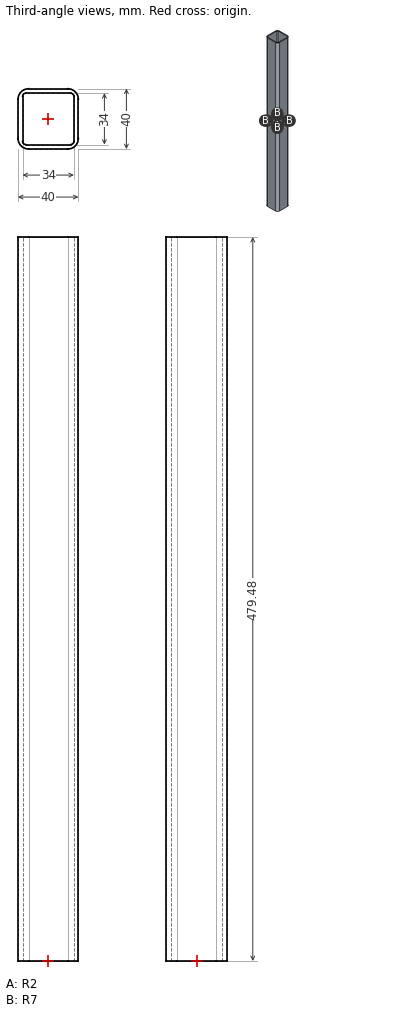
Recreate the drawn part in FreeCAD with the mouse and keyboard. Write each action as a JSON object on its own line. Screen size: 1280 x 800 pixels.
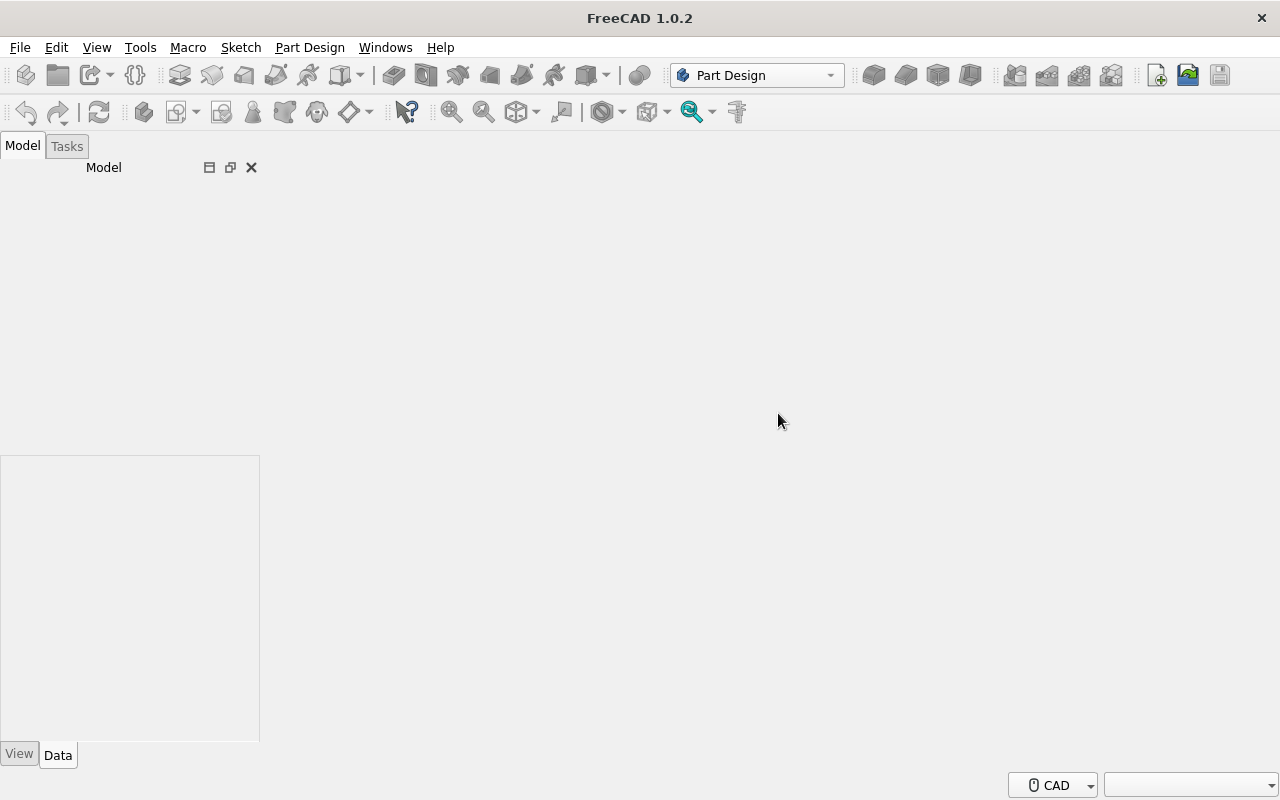
{"action": "key", "text": "ctrl+n"}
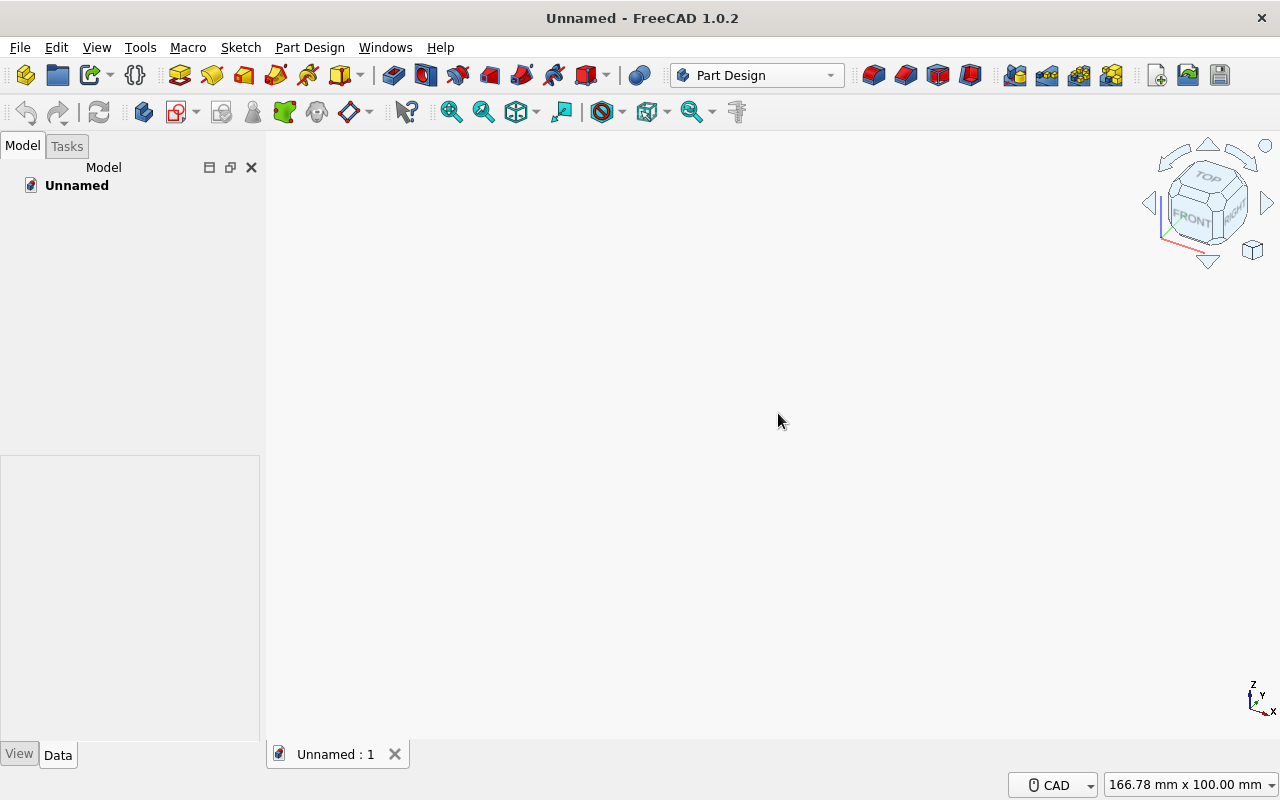
{"action": "left_click", "coordinate": [176, 112]}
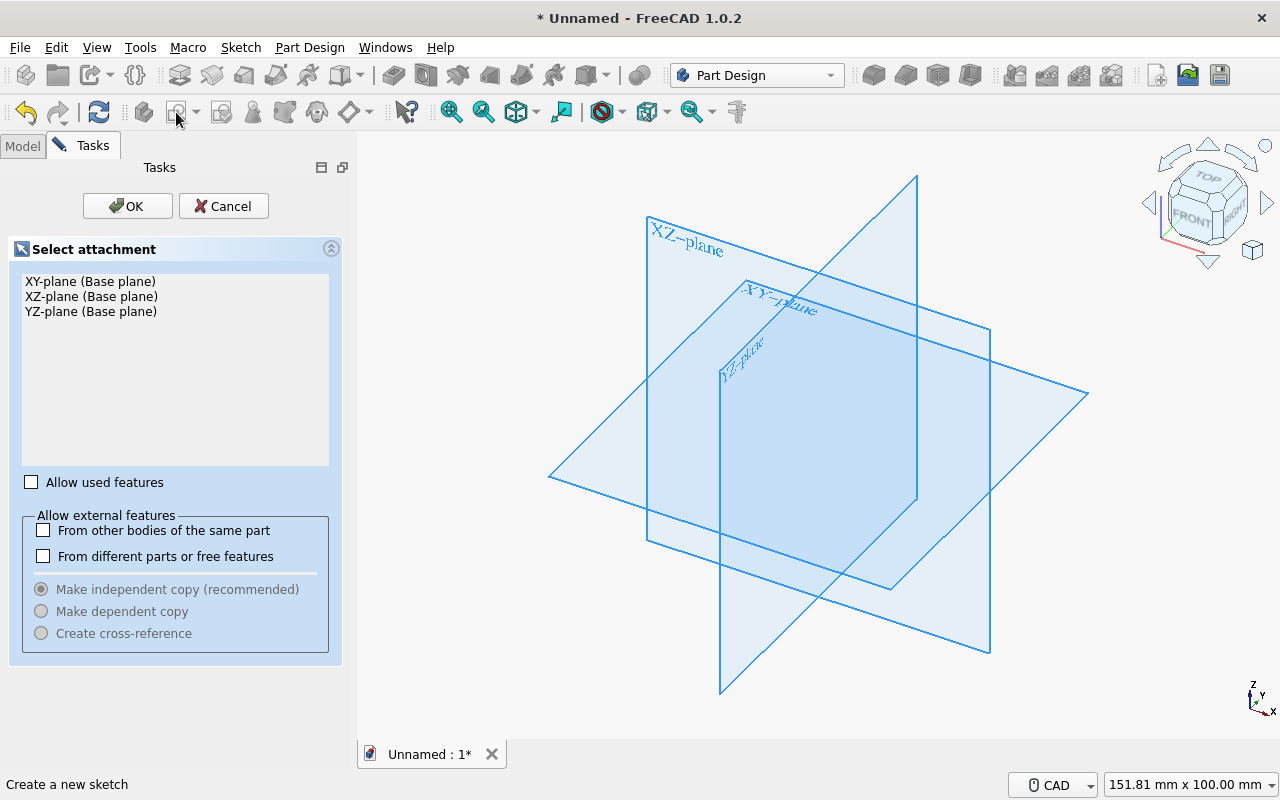
{"action": "left_click", "coordinate": [82, 282]}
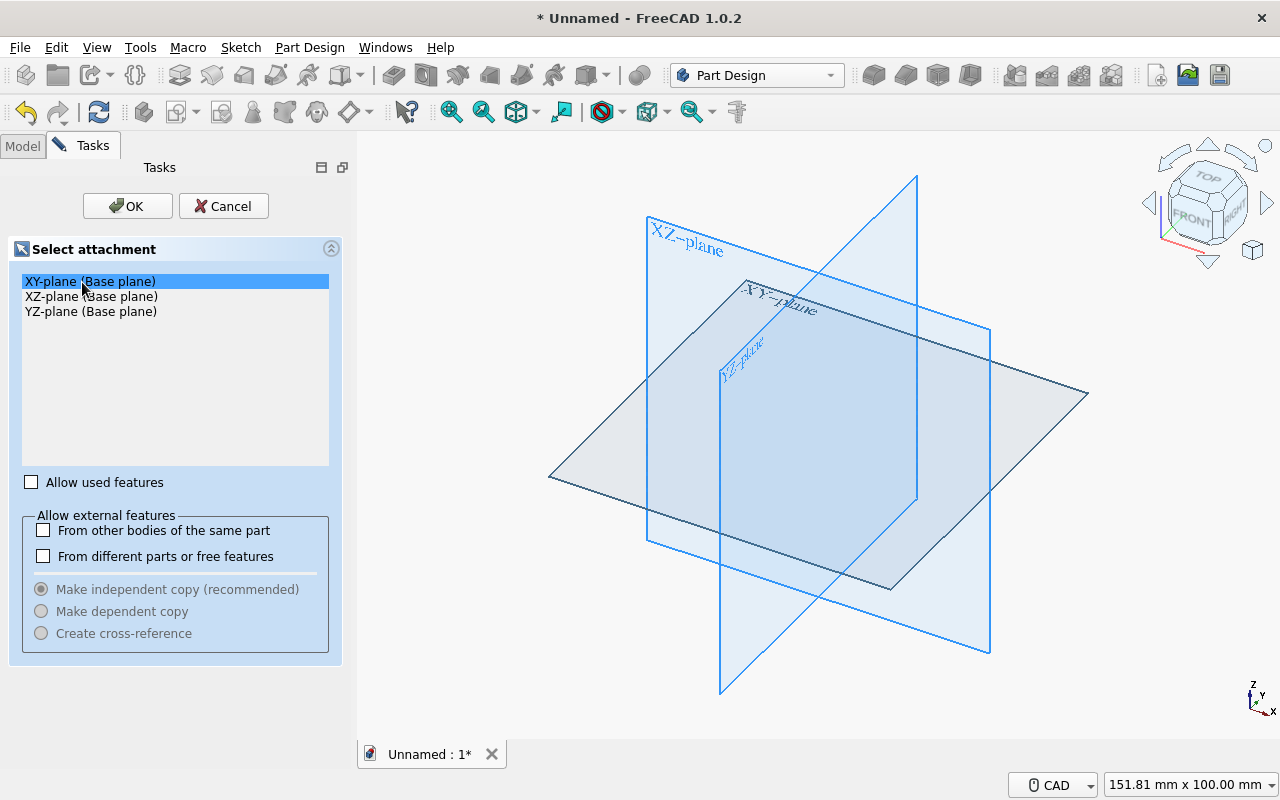
{"action": "left_click", "coordinate": [128, 206]}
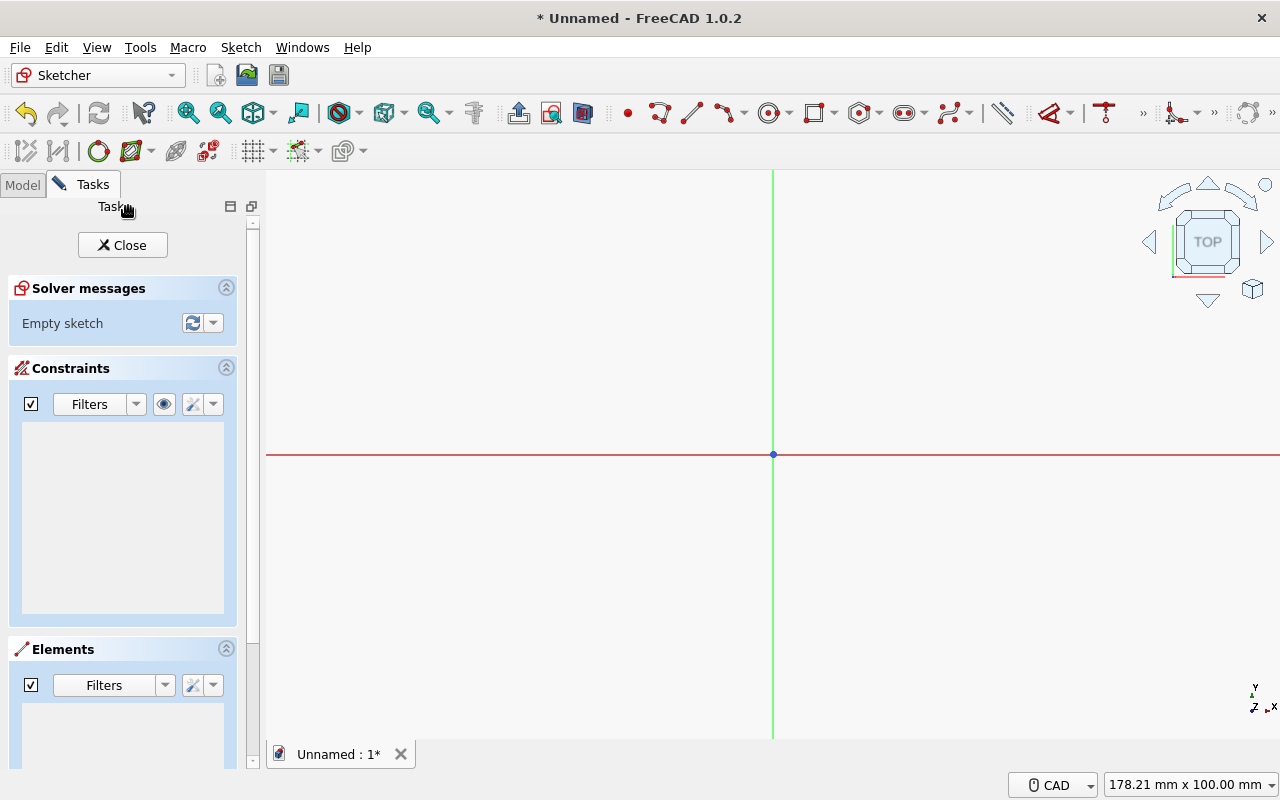
{"action": "scroll", "coordinate": [912, 455], "scroll_direction": "up", "scroll_amount": 2}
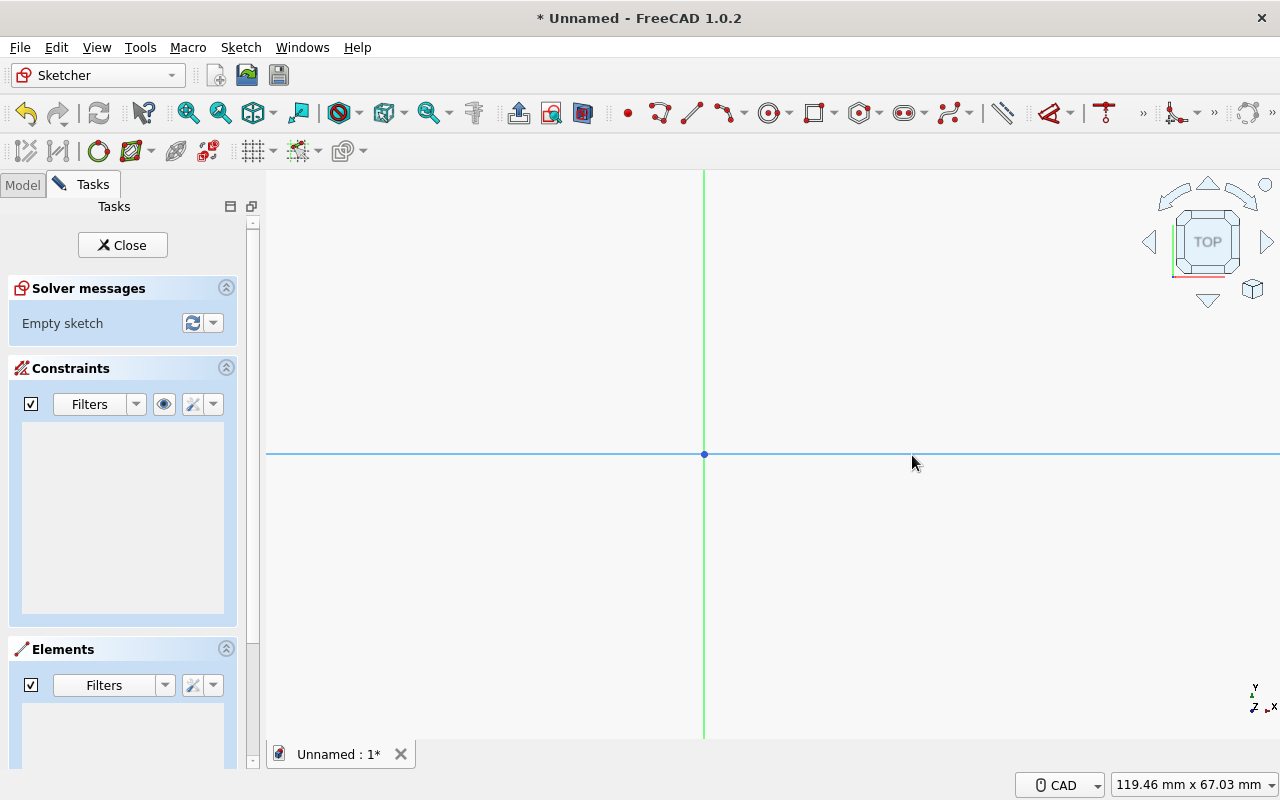
{"action": "left_click", "coordinate": [836, 114]}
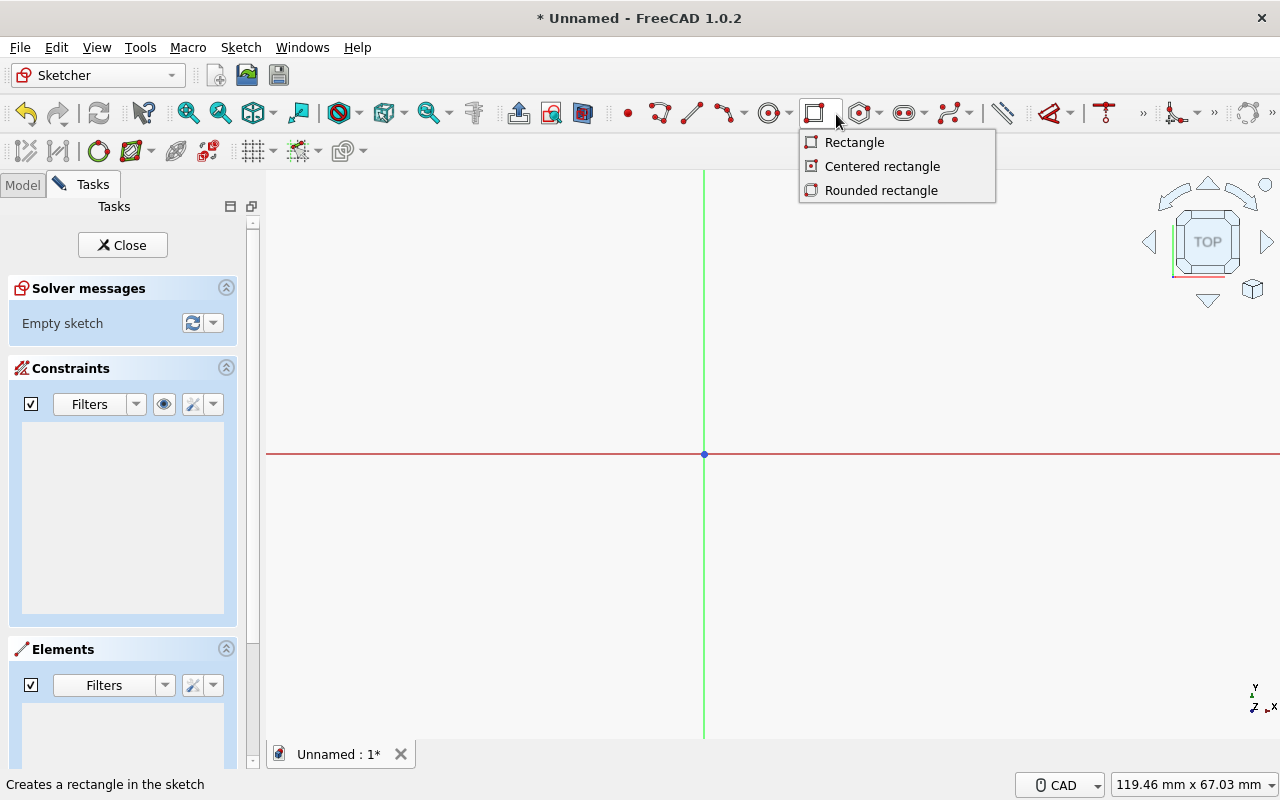
{"action": "left_click", "coordinate": [898, 166]}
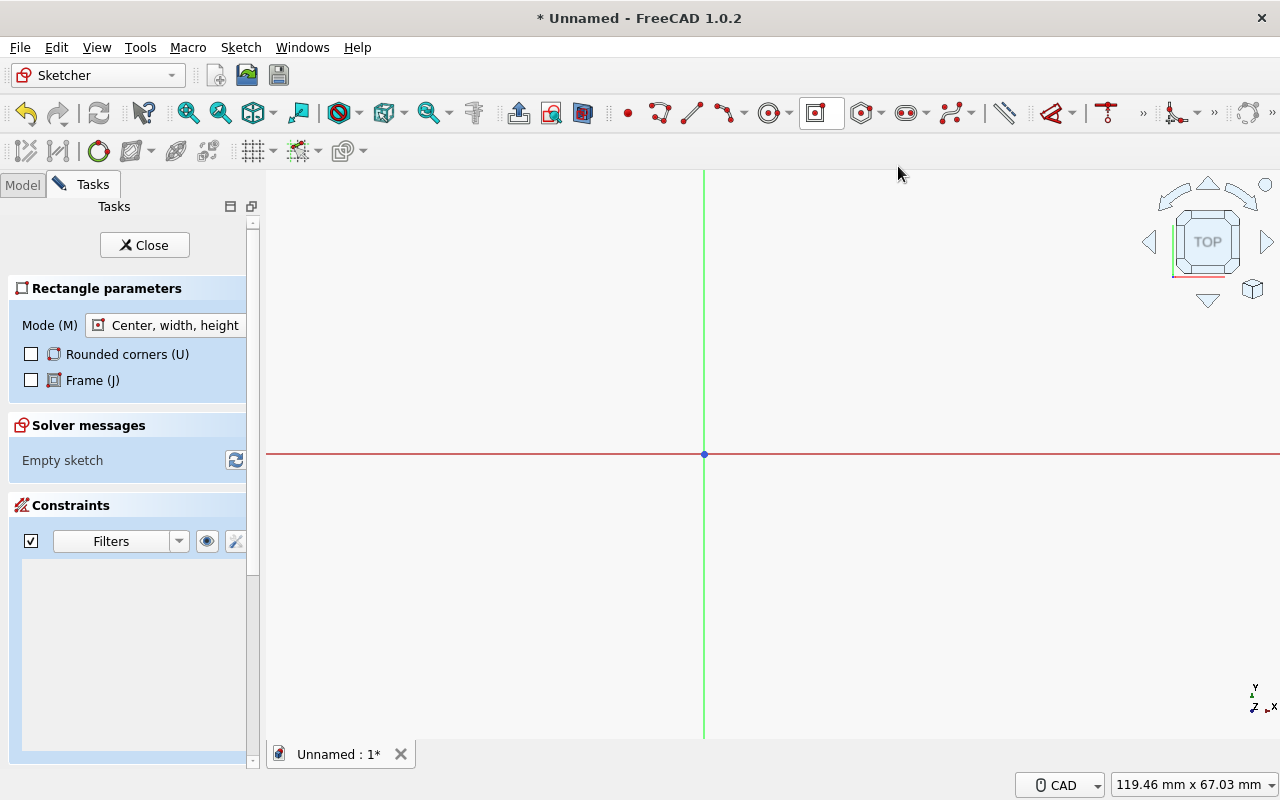
{"action": "left_click", "coordinate": [704, 454]}
{"action": "left_click", "coordinate": [874, 284]}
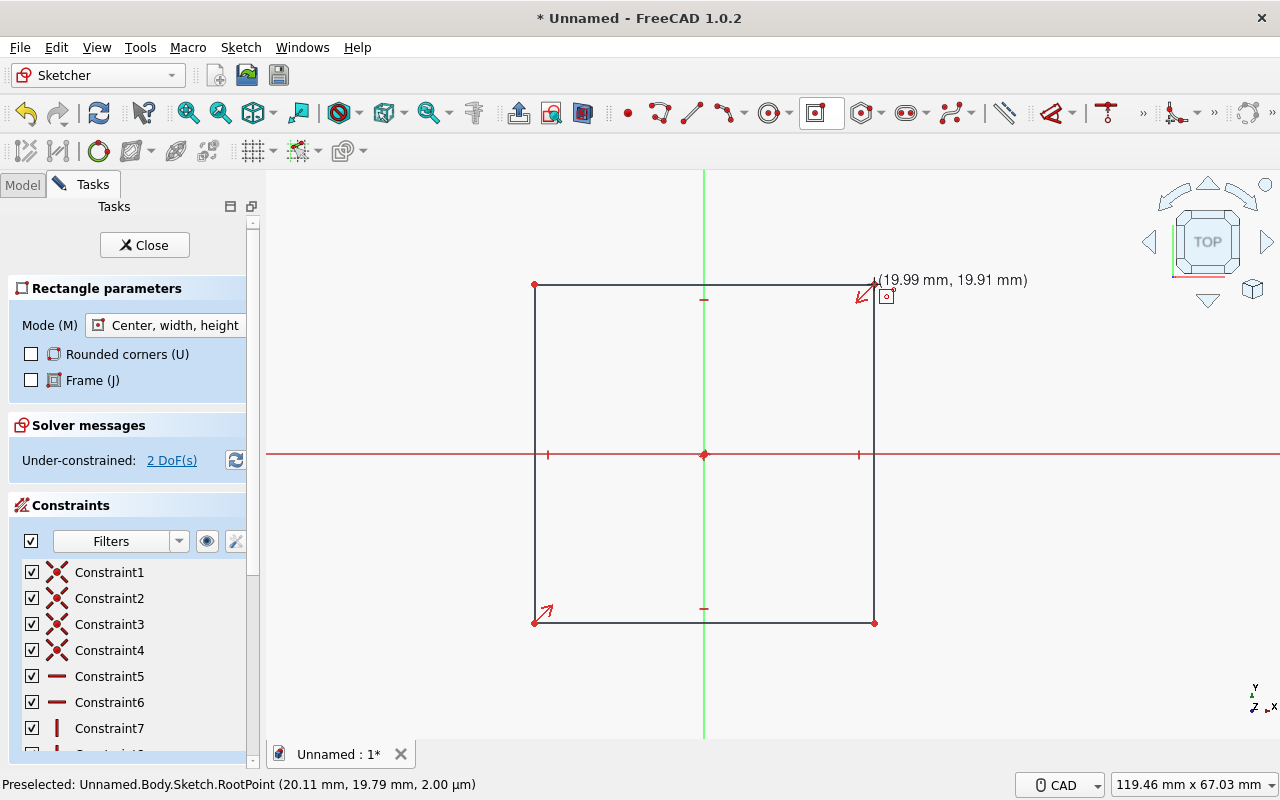
{"action": "left_click", "coordinate": [704, 454]}
{"action": "left_click", "coordinate": [849, 310]}
{"action": "key", "text": "Escape"}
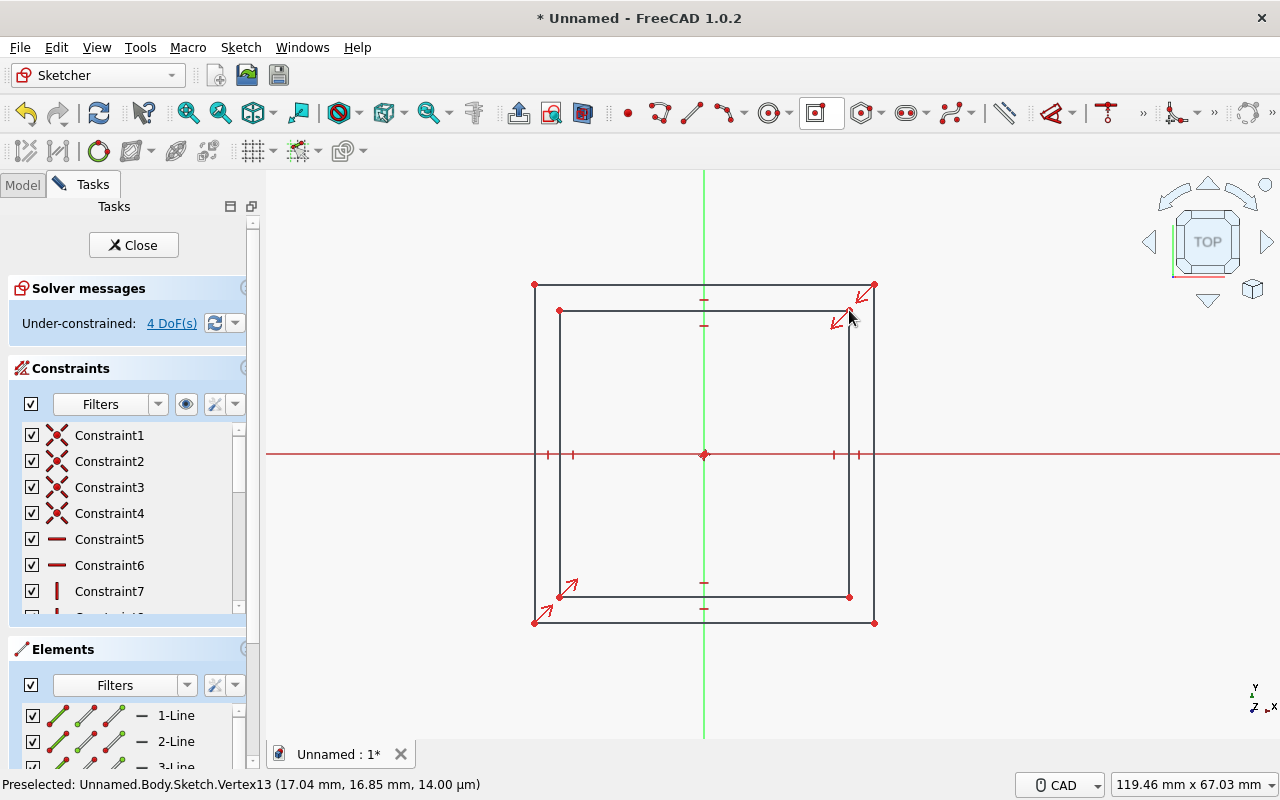
{"action": "left_click", "coordinate": [636, 623]}